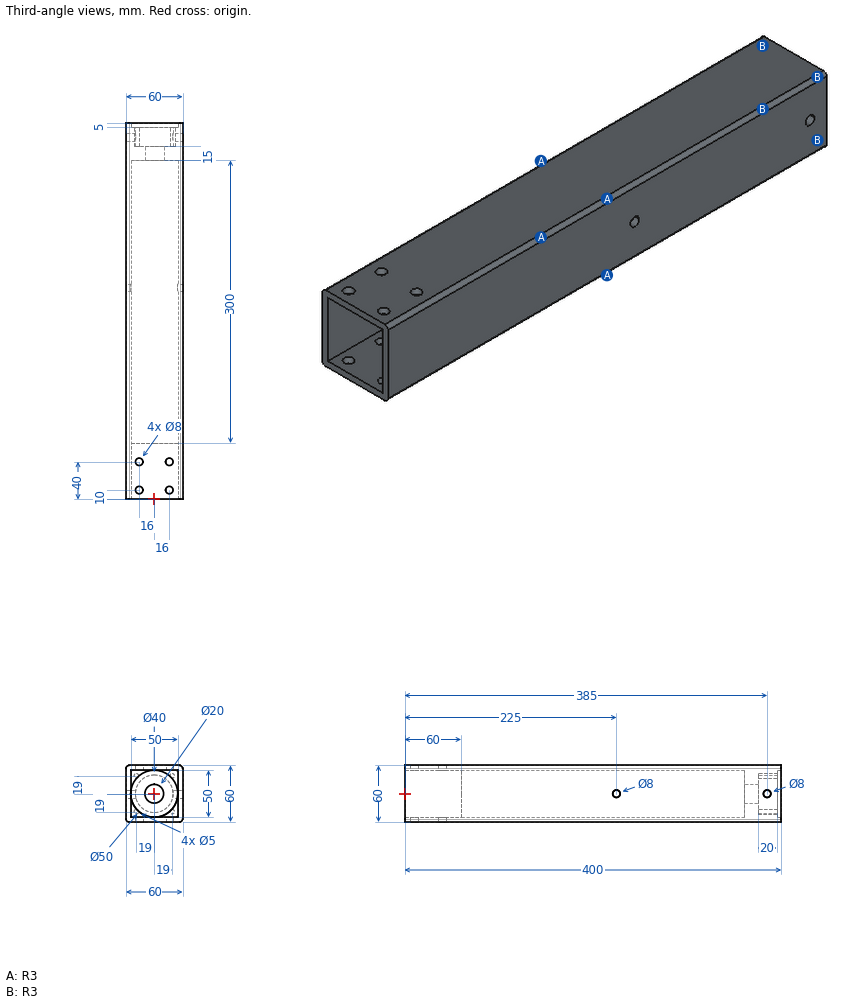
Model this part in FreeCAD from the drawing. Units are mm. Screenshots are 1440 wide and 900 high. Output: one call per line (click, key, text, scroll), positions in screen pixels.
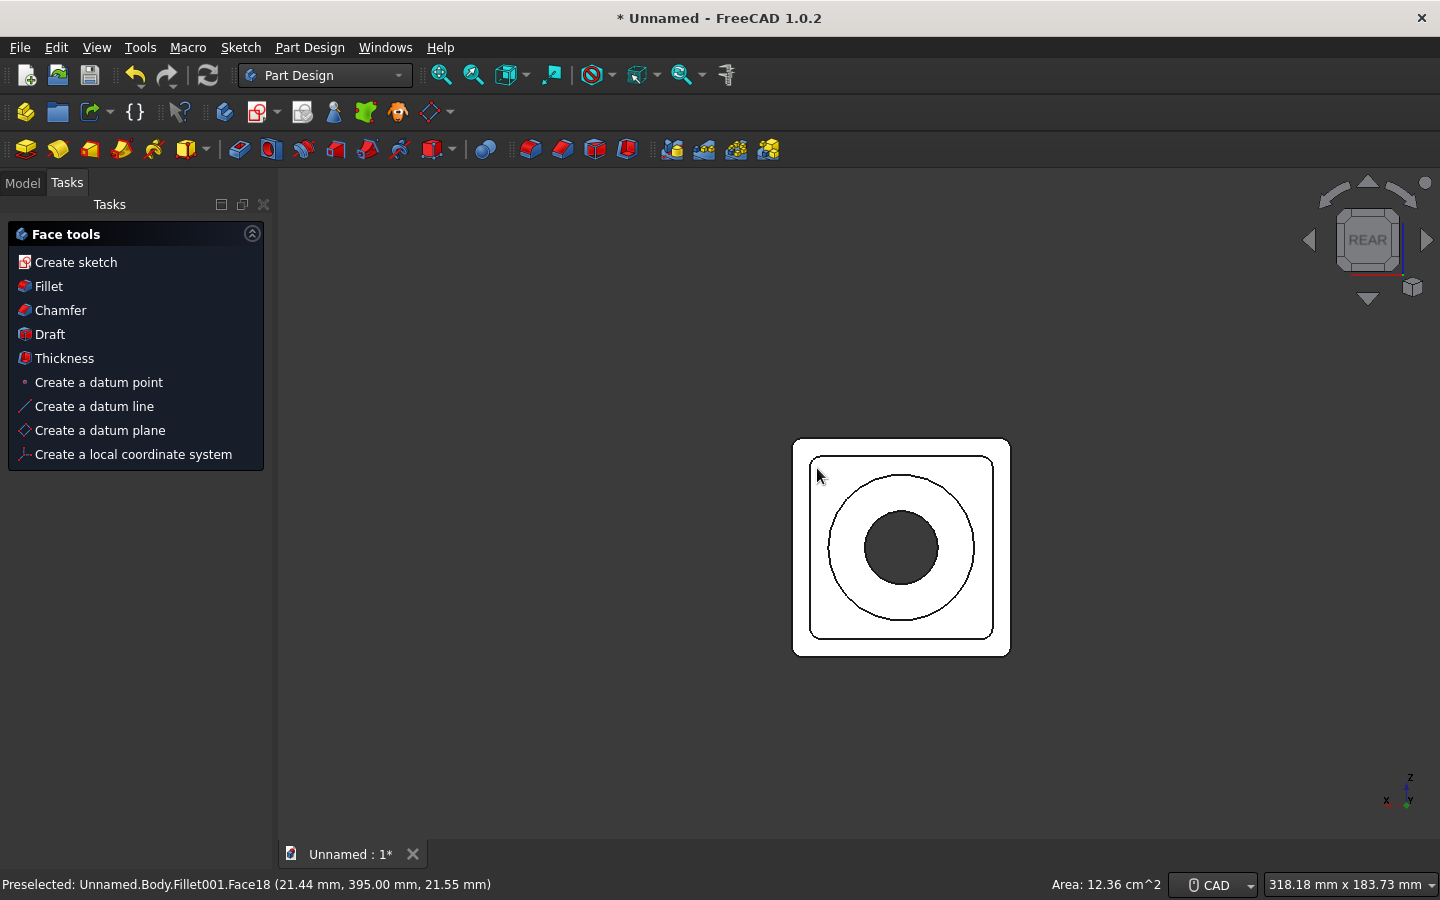
click(258, 112)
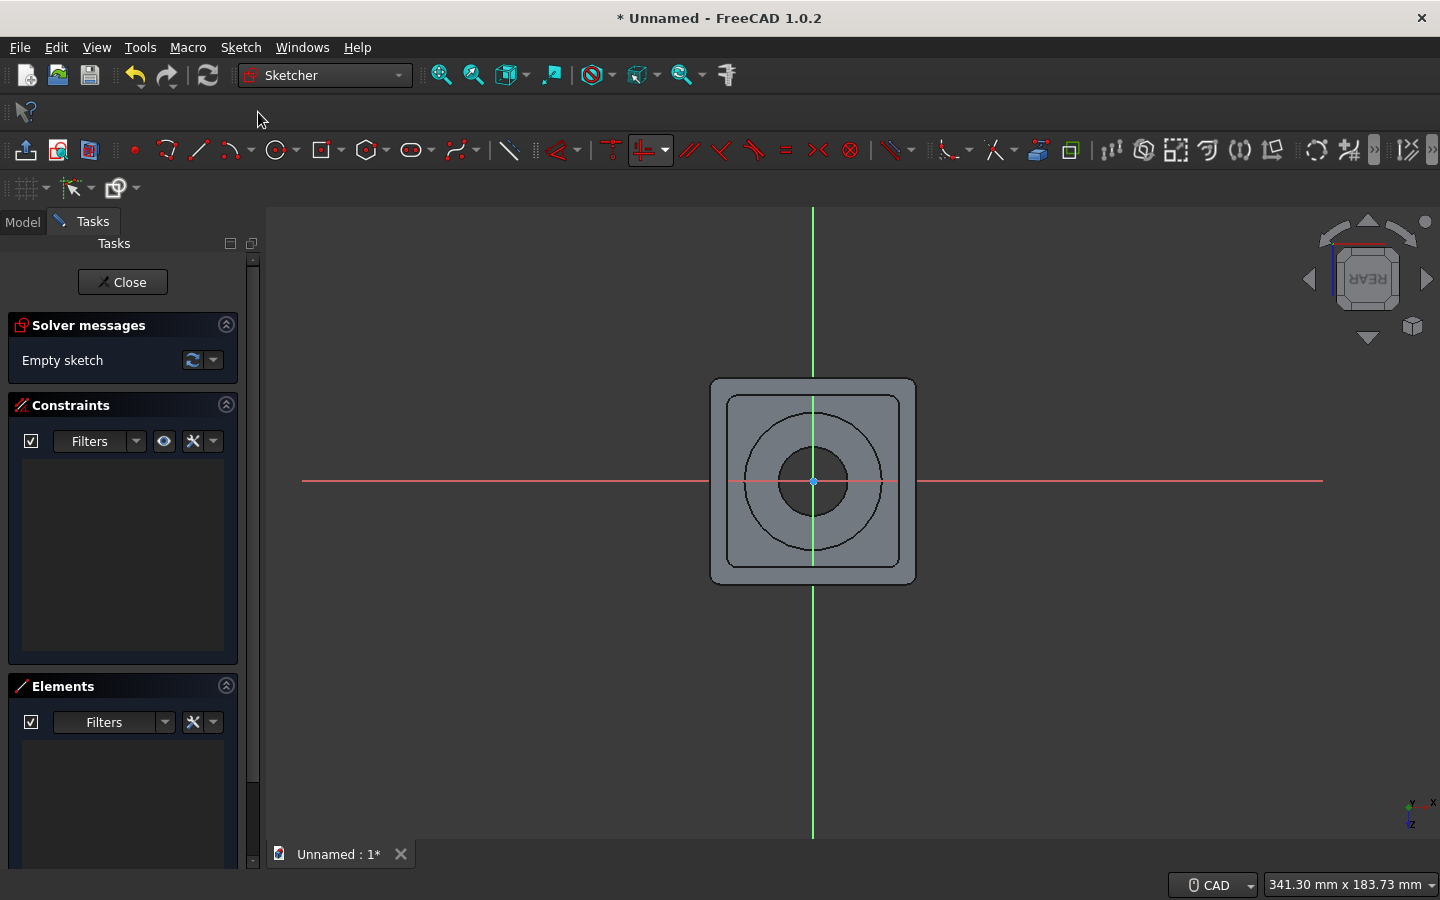
scroll(830, 457, up, 5)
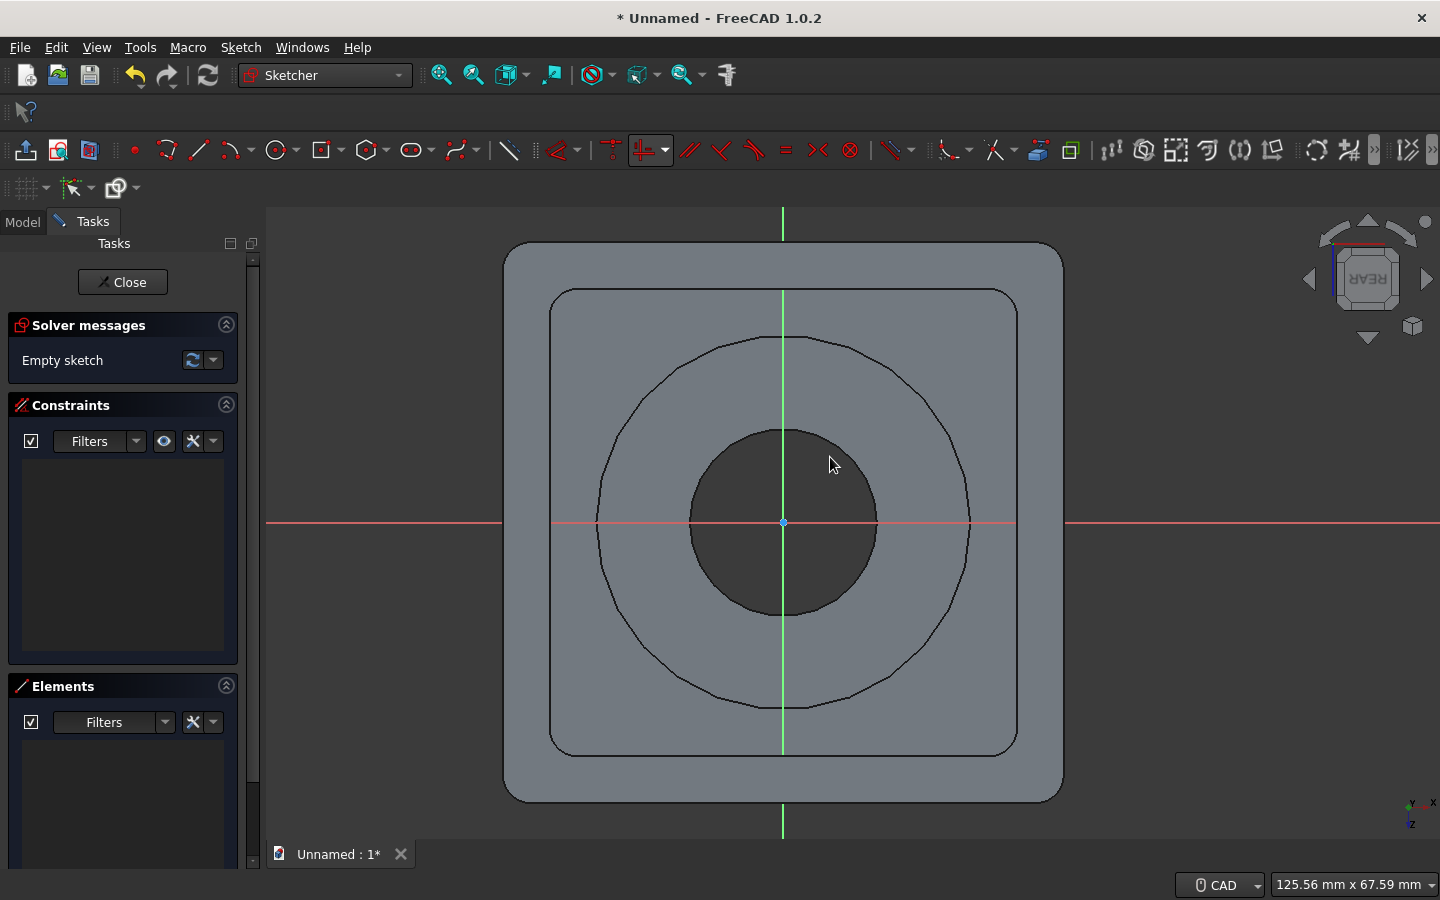
click(276, 150)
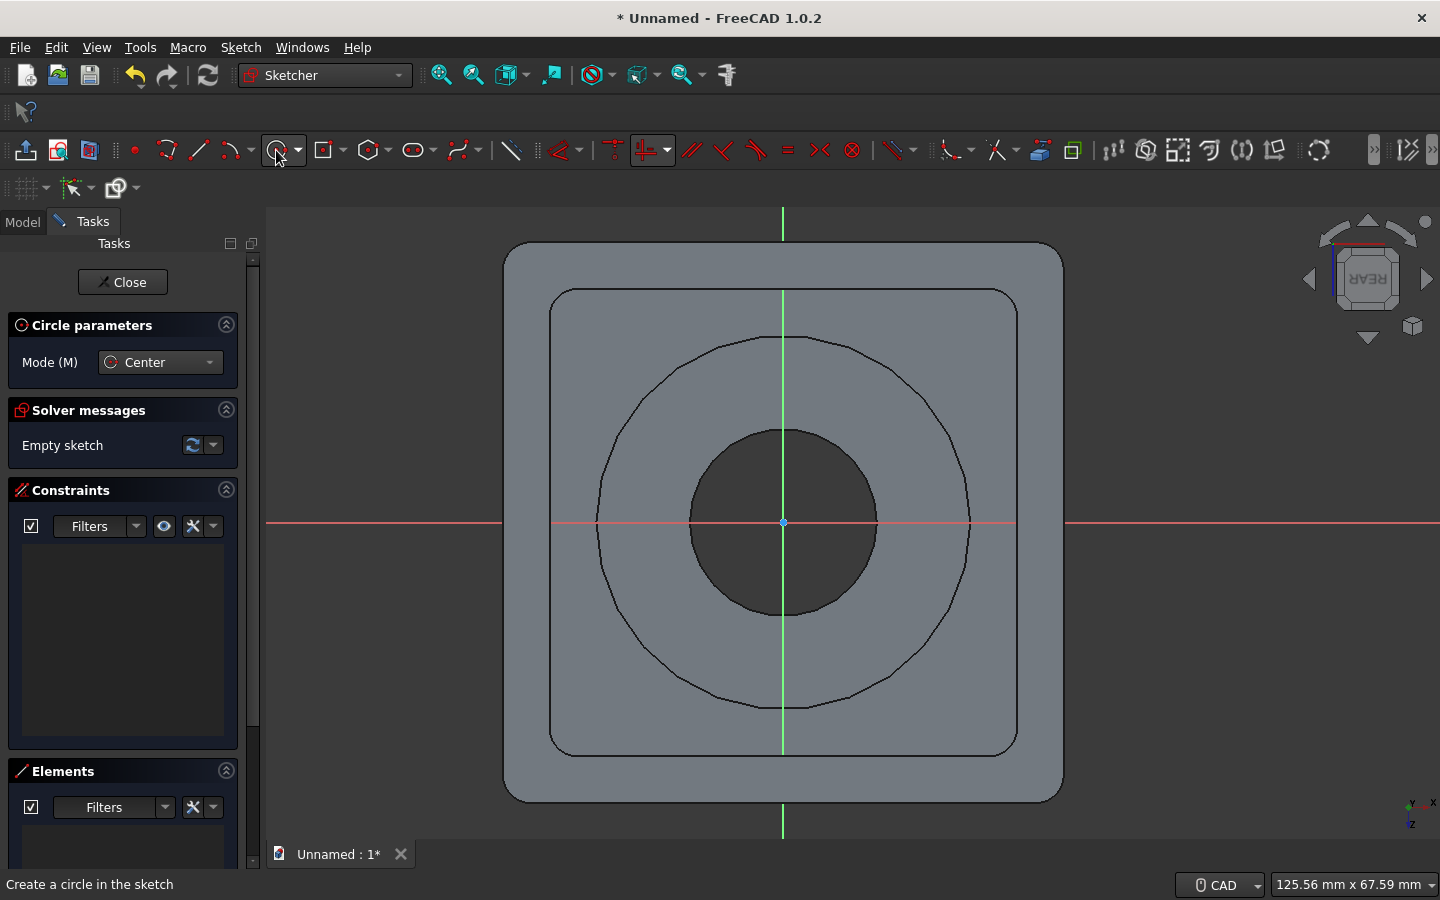
click(606, 345)
move(622, 328)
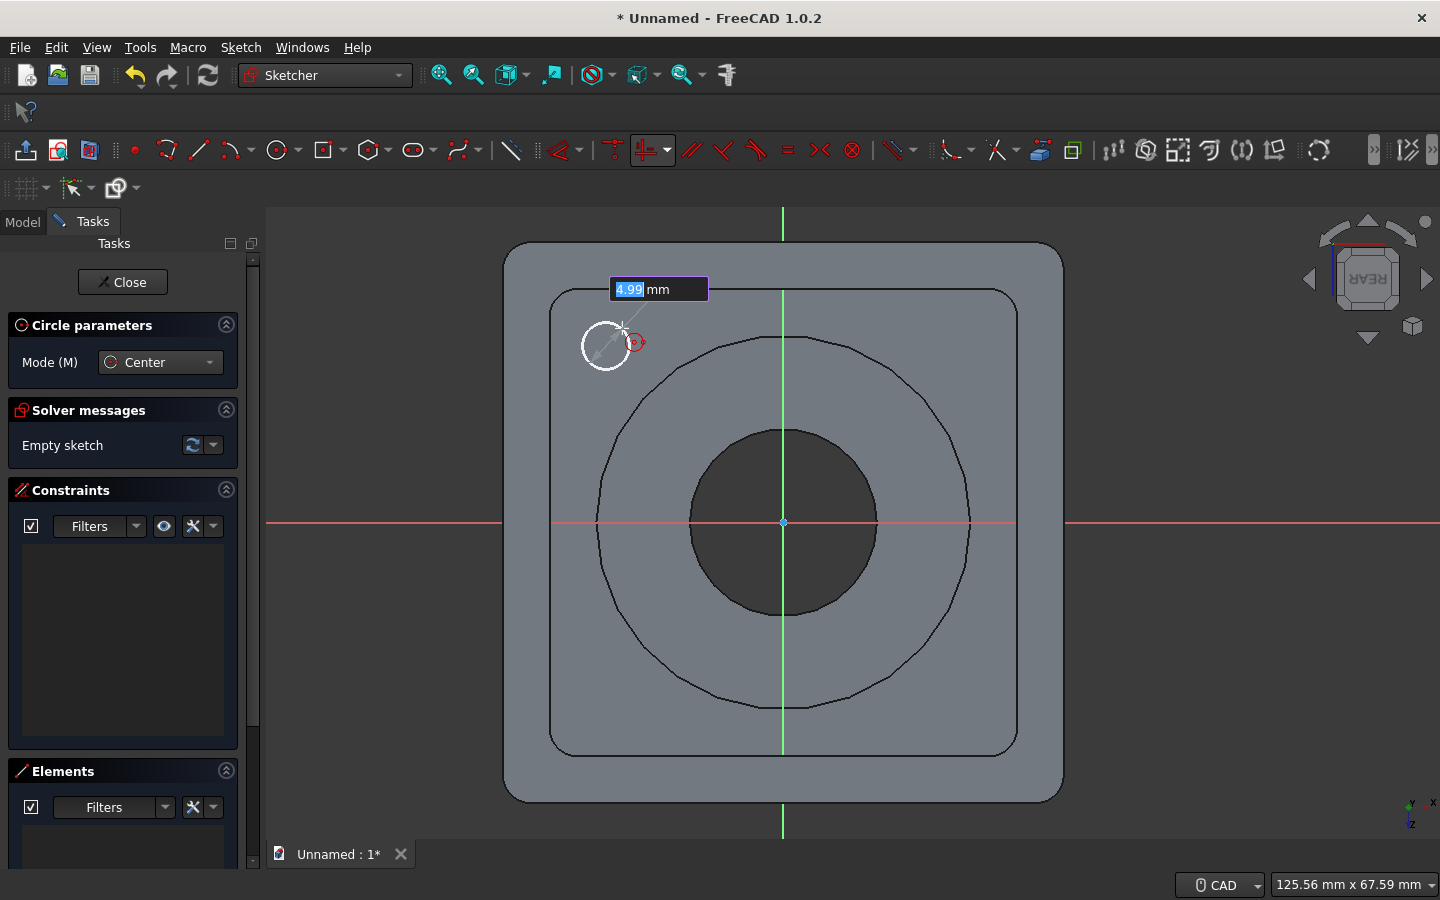
text(5)
key(Return)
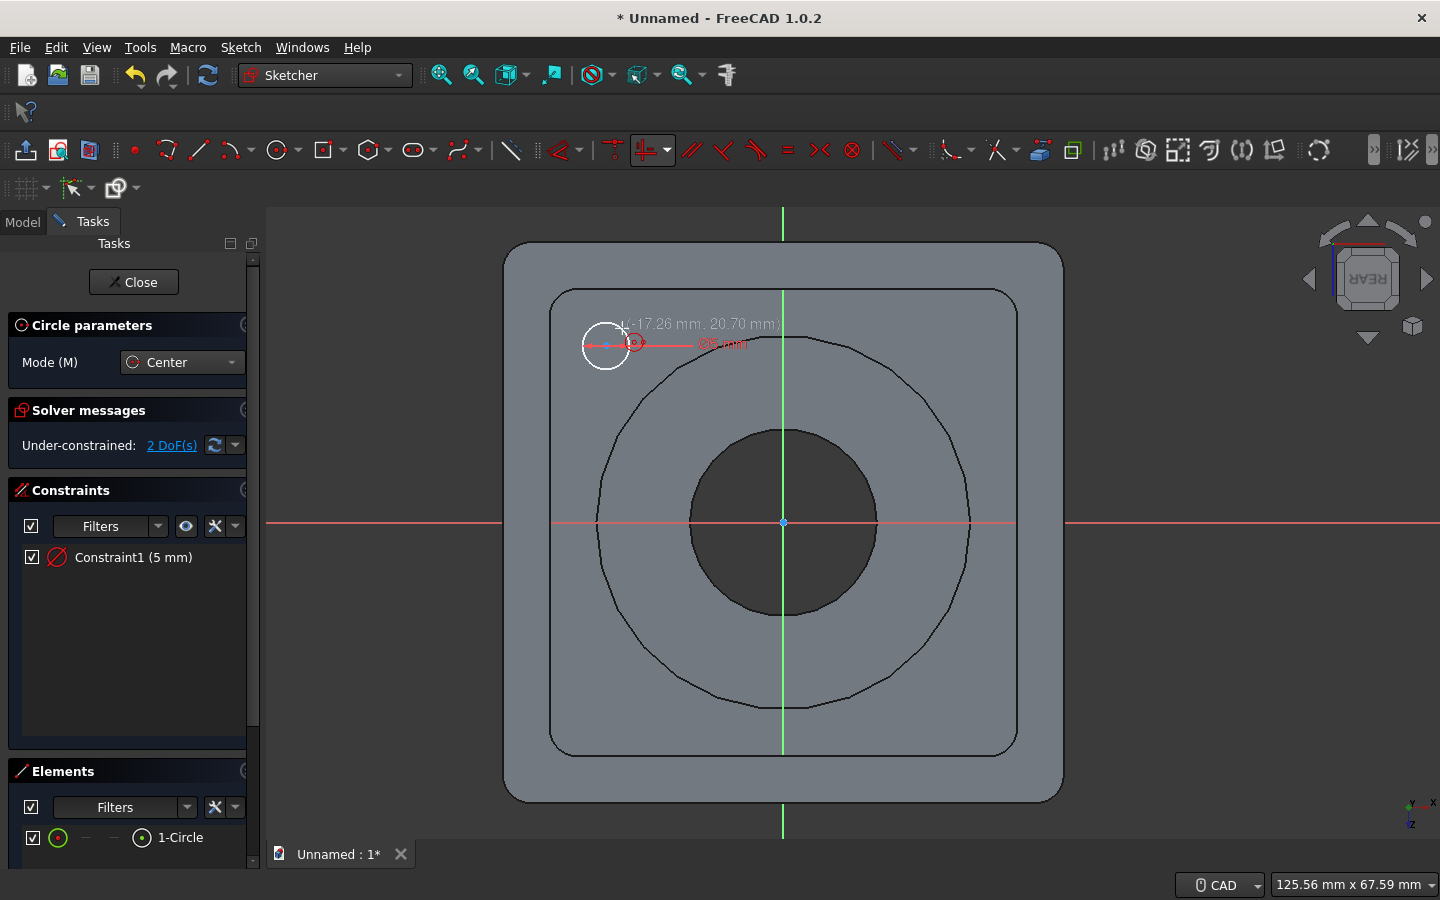
click(961, 345)
move(978, 328)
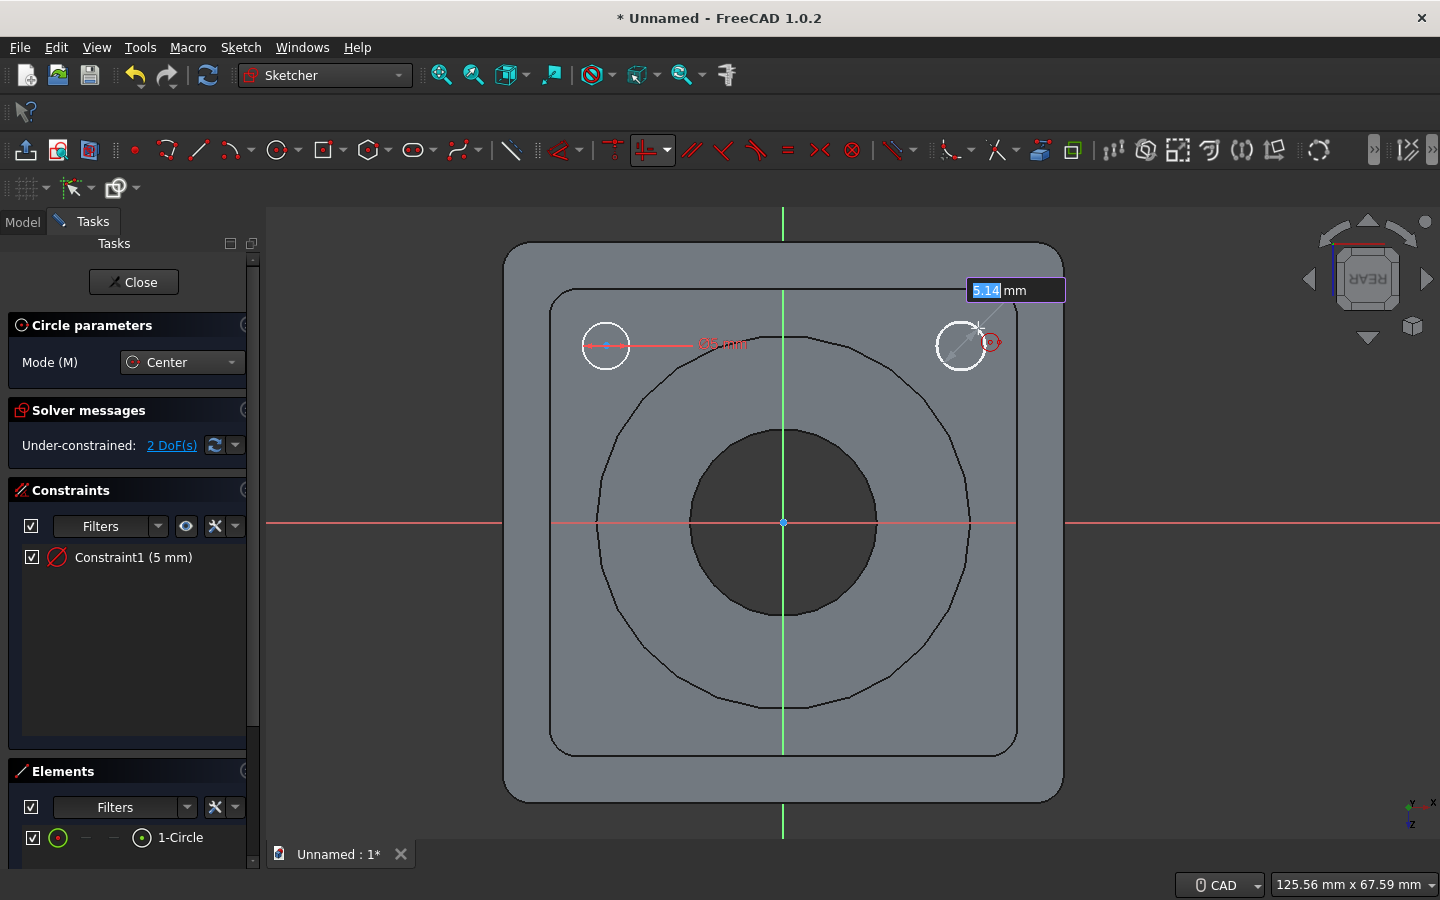
text(5)
key(Return)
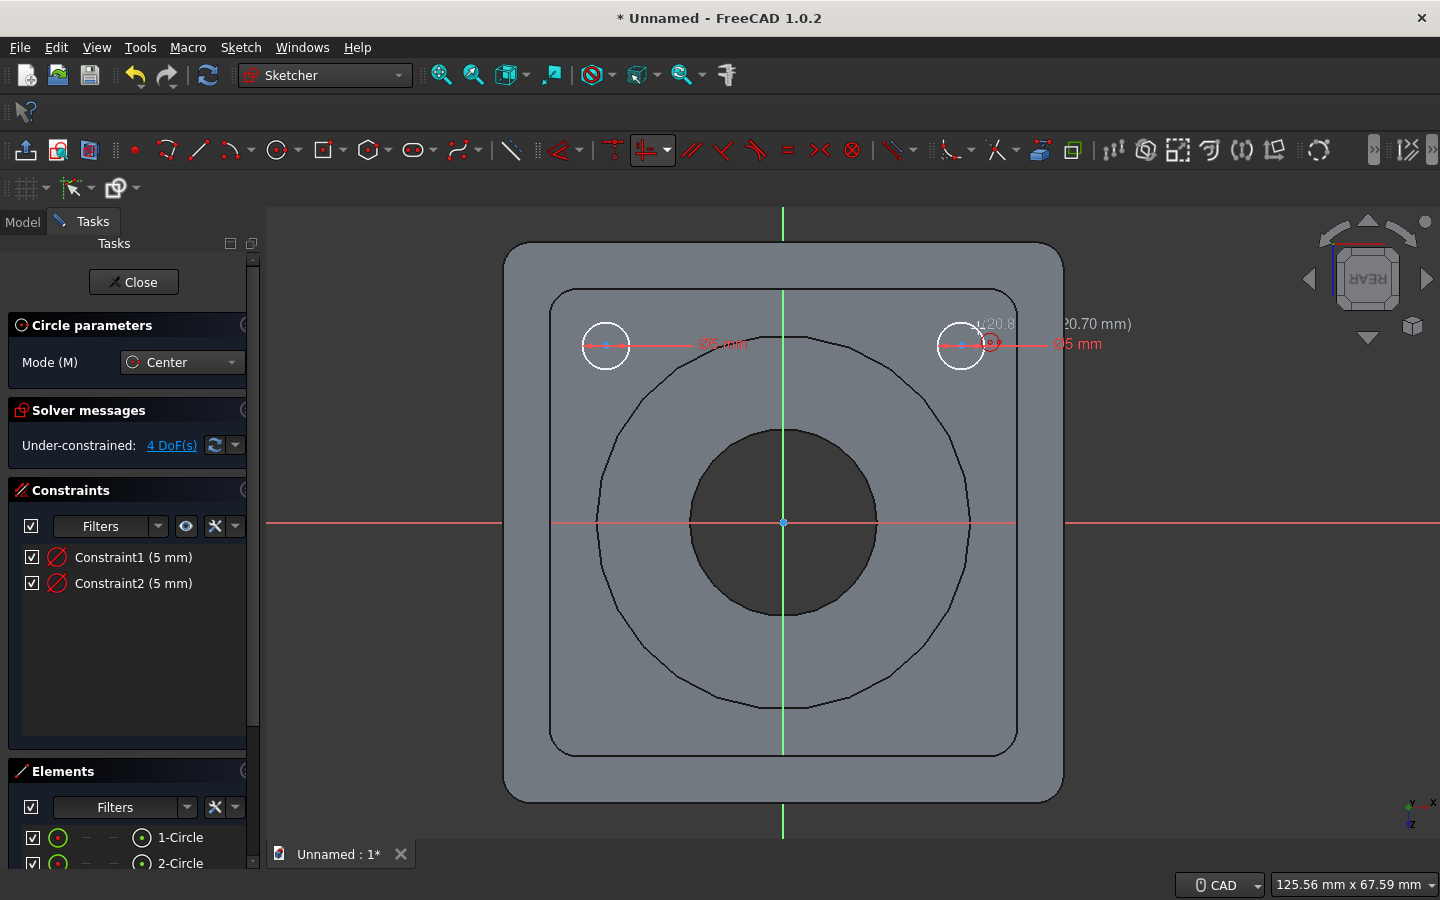
click(606, 700)
move(622, 684)